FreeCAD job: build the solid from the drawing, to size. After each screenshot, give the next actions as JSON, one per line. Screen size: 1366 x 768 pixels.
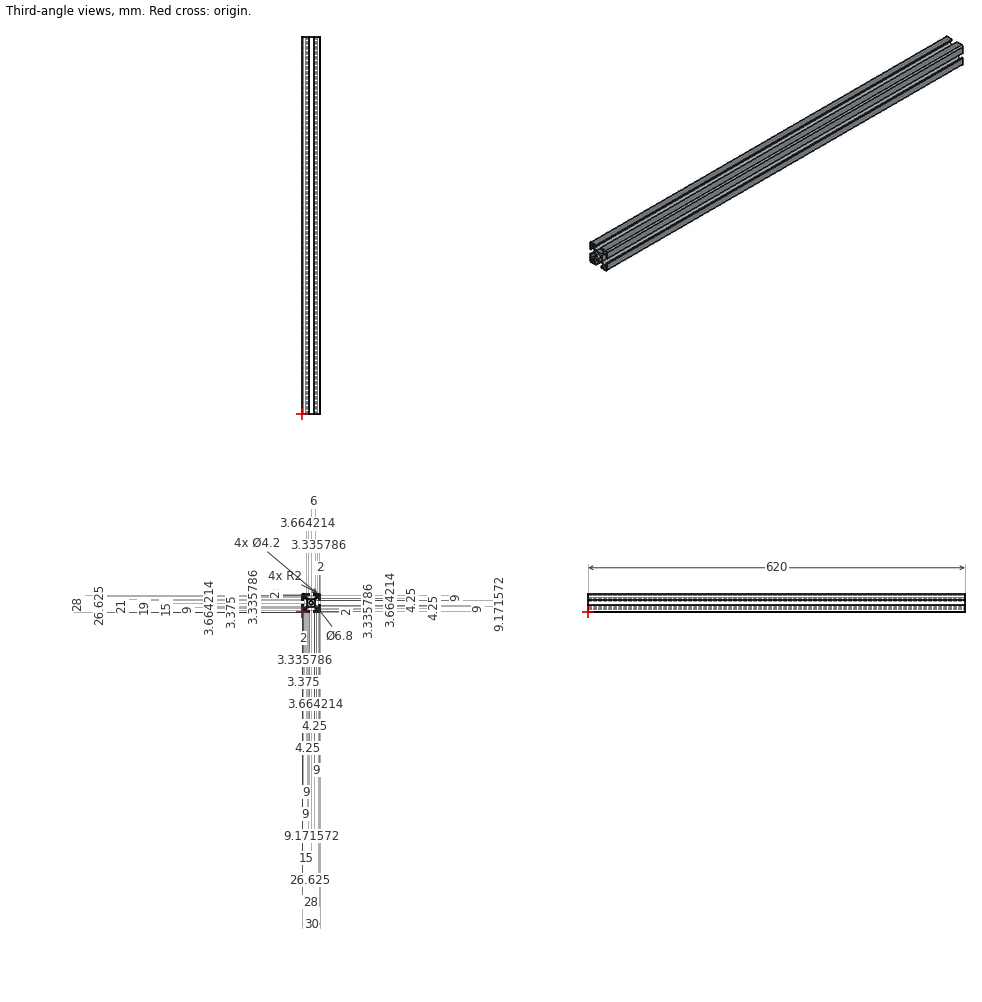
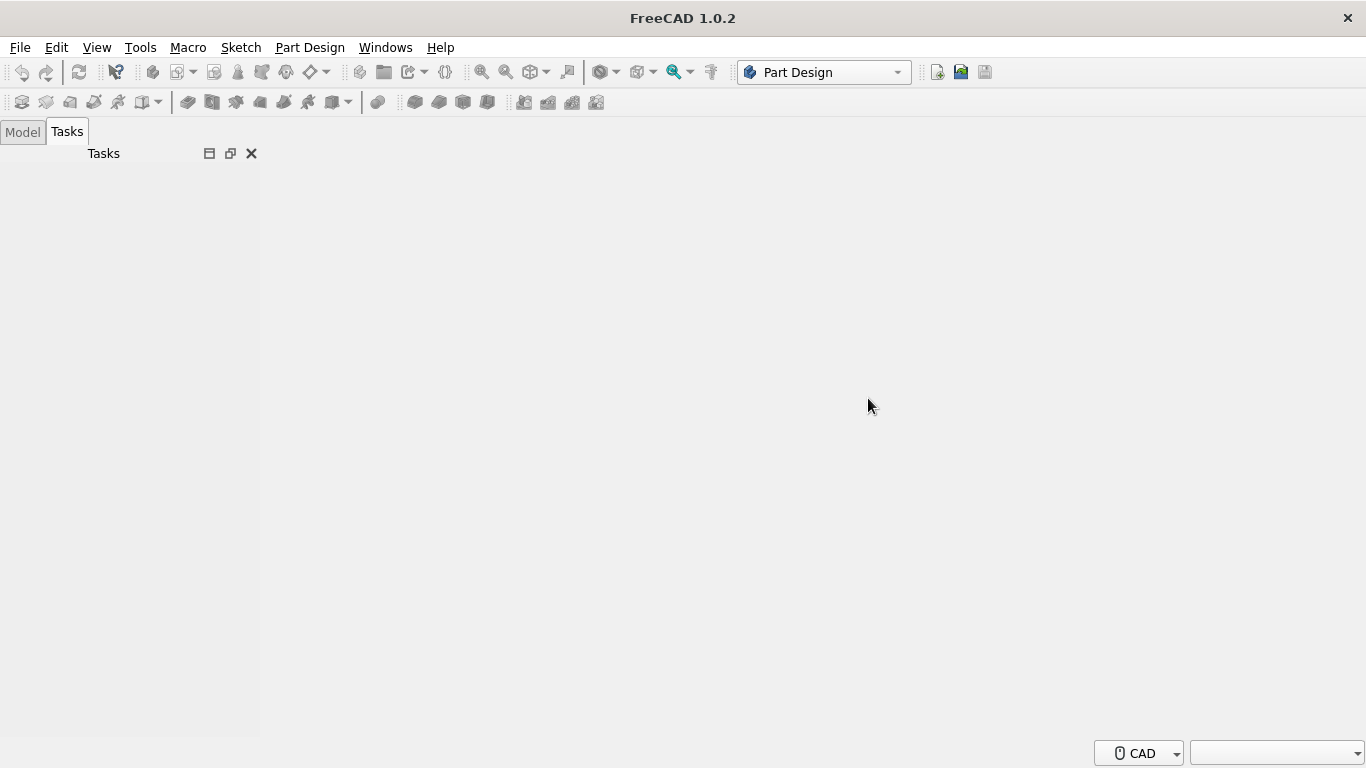
{"action": "left_click", "coordinate": [938, 72]}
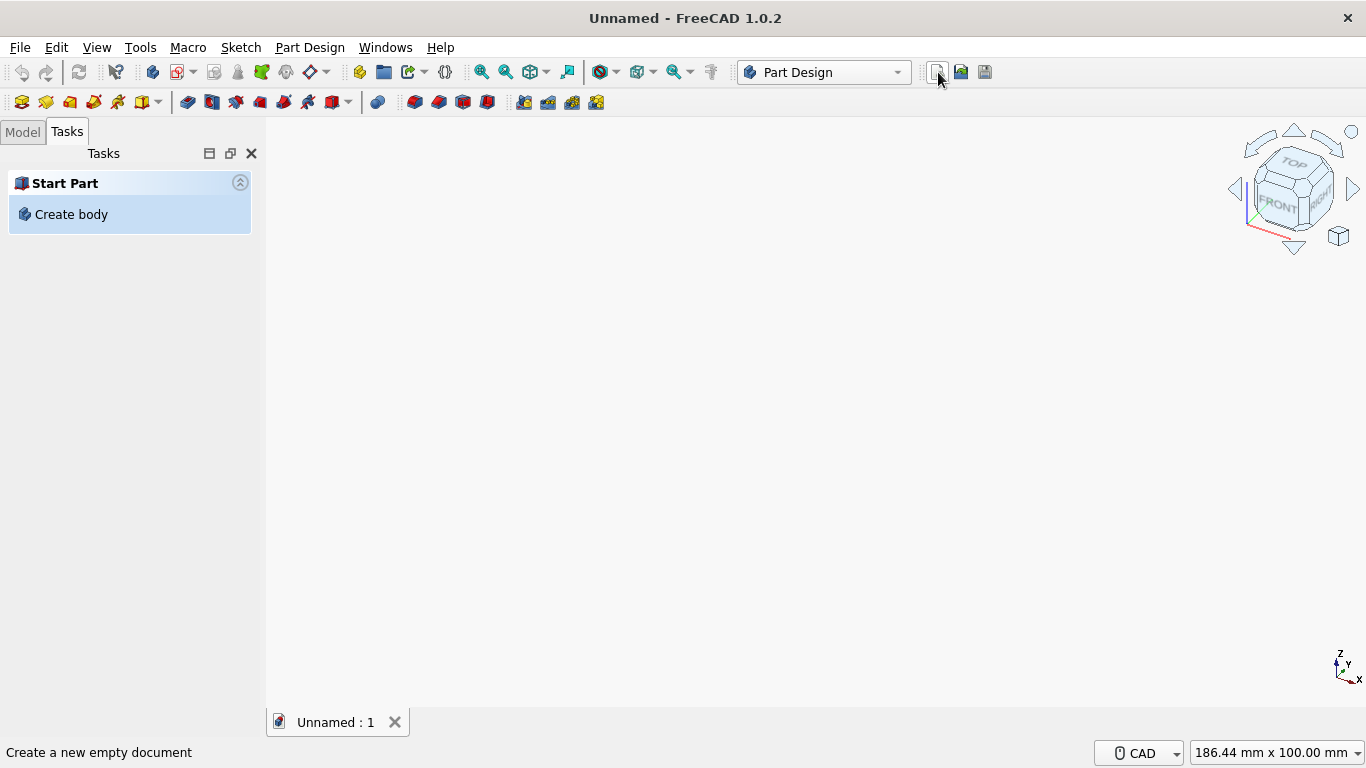
{"action": "left_click", "coordinate": [178, 72]}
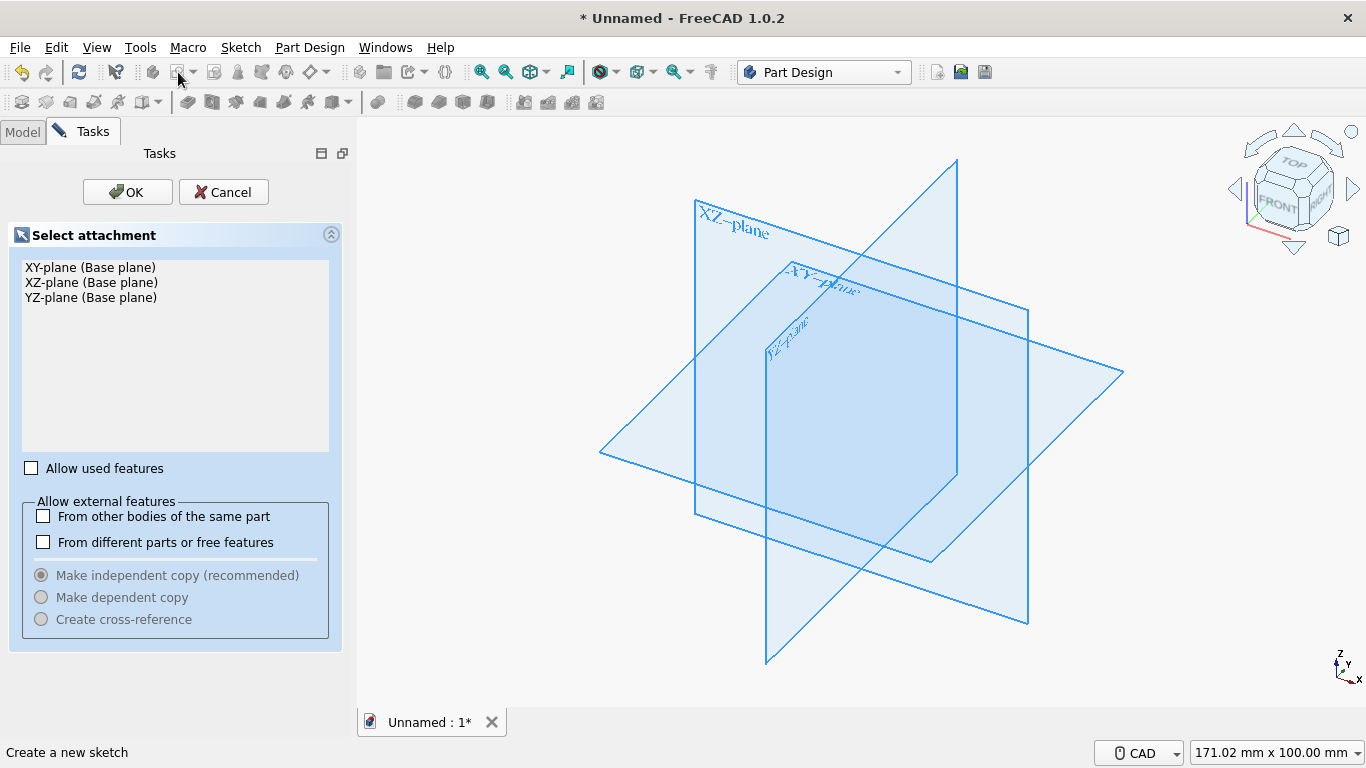
{"action": "left_click", "coordinate": [82, 282]}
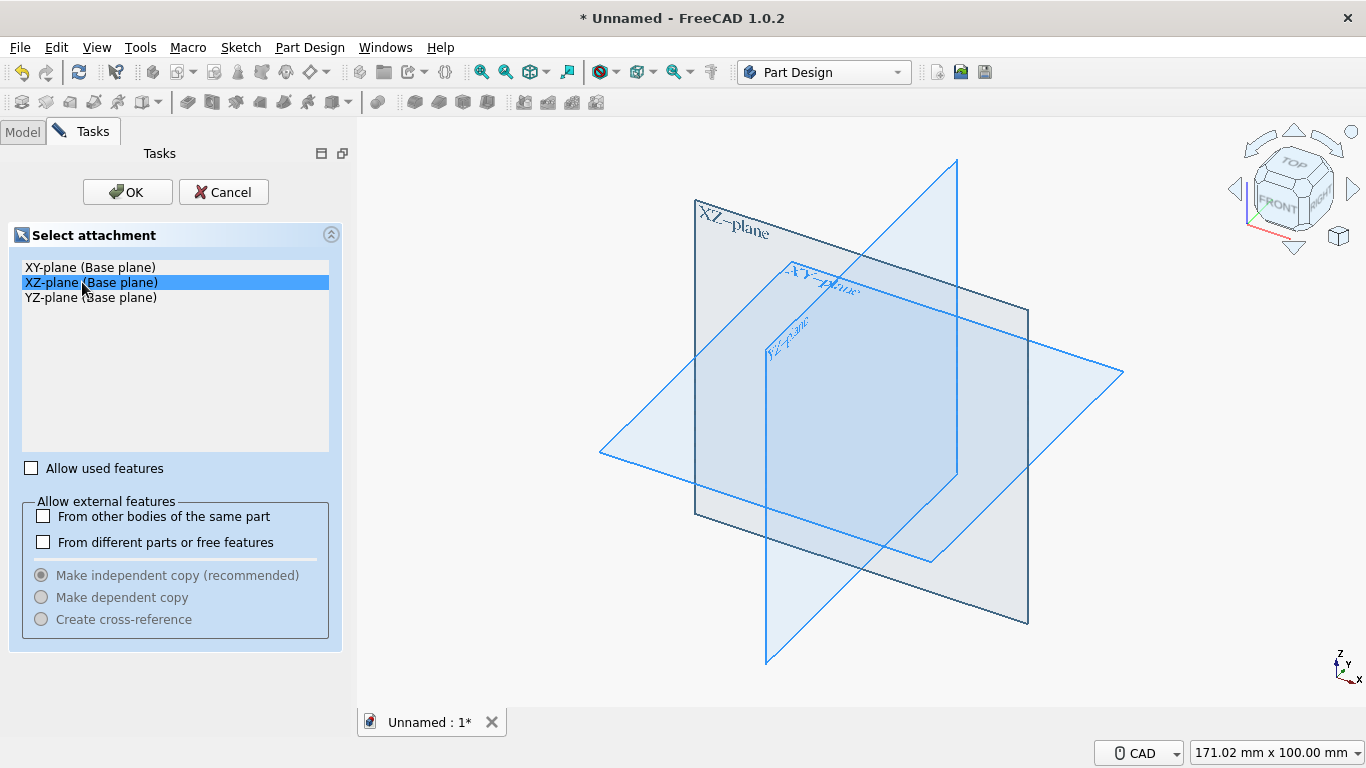
{"action": "left_click", "coordinate": [128, 192]}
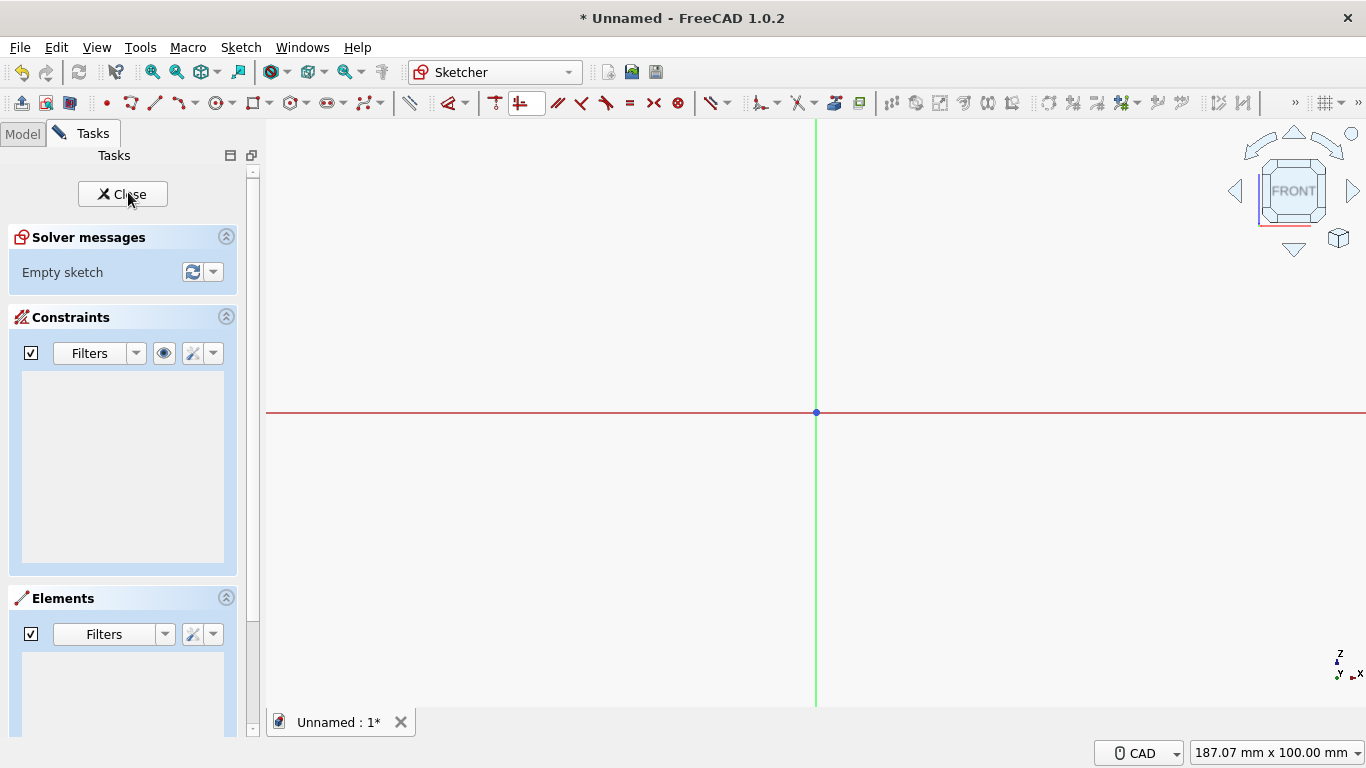
{"action": "scroll", "coordinate": [1032, 253], "scroll_direction": "up", "scroll_amount": 4}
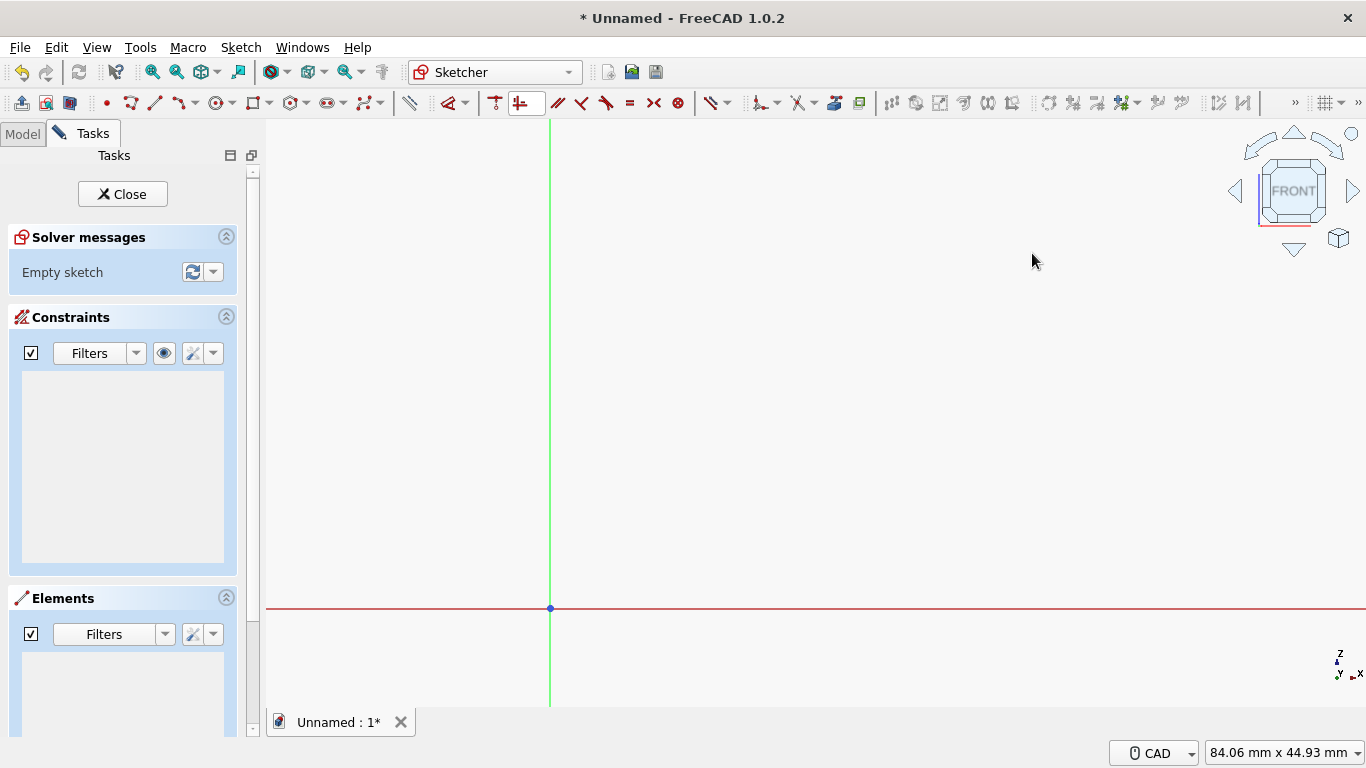
{"action": "left_click", "coordinate": [132, 104]}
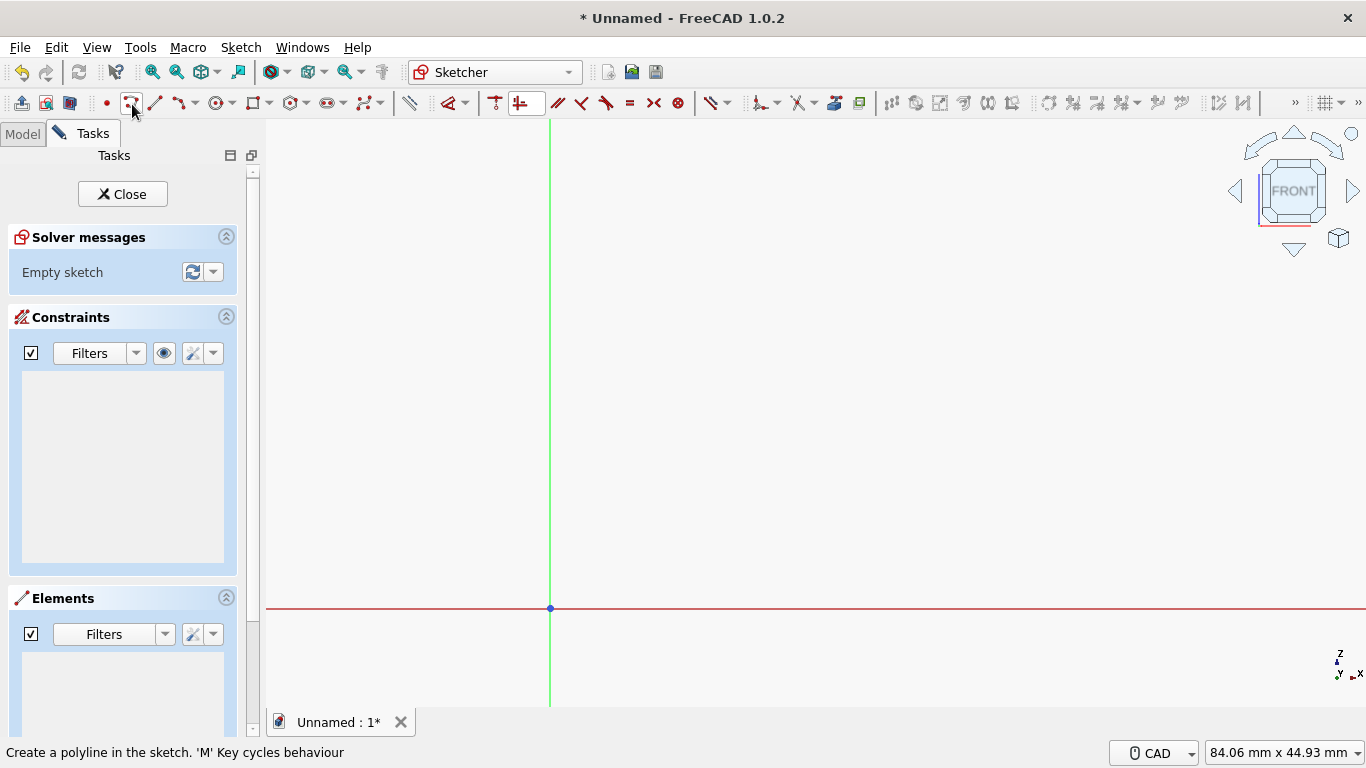
{"action": "left_click", "coordinate": [943, 242]}
{"action": "left_click", "coordinate": [943, 360]}
{"action": "left_click", "coordinate": [917, 360]}
{"action": "left_click", "coordinate": [917, 305]}
{"action": "left_click", "coordinate": [873, 305]}
{"action": "left_click", "coordinate": [825, 353]}
{"action": "left_click", "coordinate": [825, 473]}
{"action": "left_click", "coordinate": [873, 520]}
{"action": "left_click", "coordinate": [917, 520]}
{"action": "left_click", "coordinate": [917, 465]}
{"action": "left_click", "coordinate": [943, 465]}
{"action": "left_click", "coordinate": [943, 583]}
{"action": "right_click", "coordinate": [943, 583]}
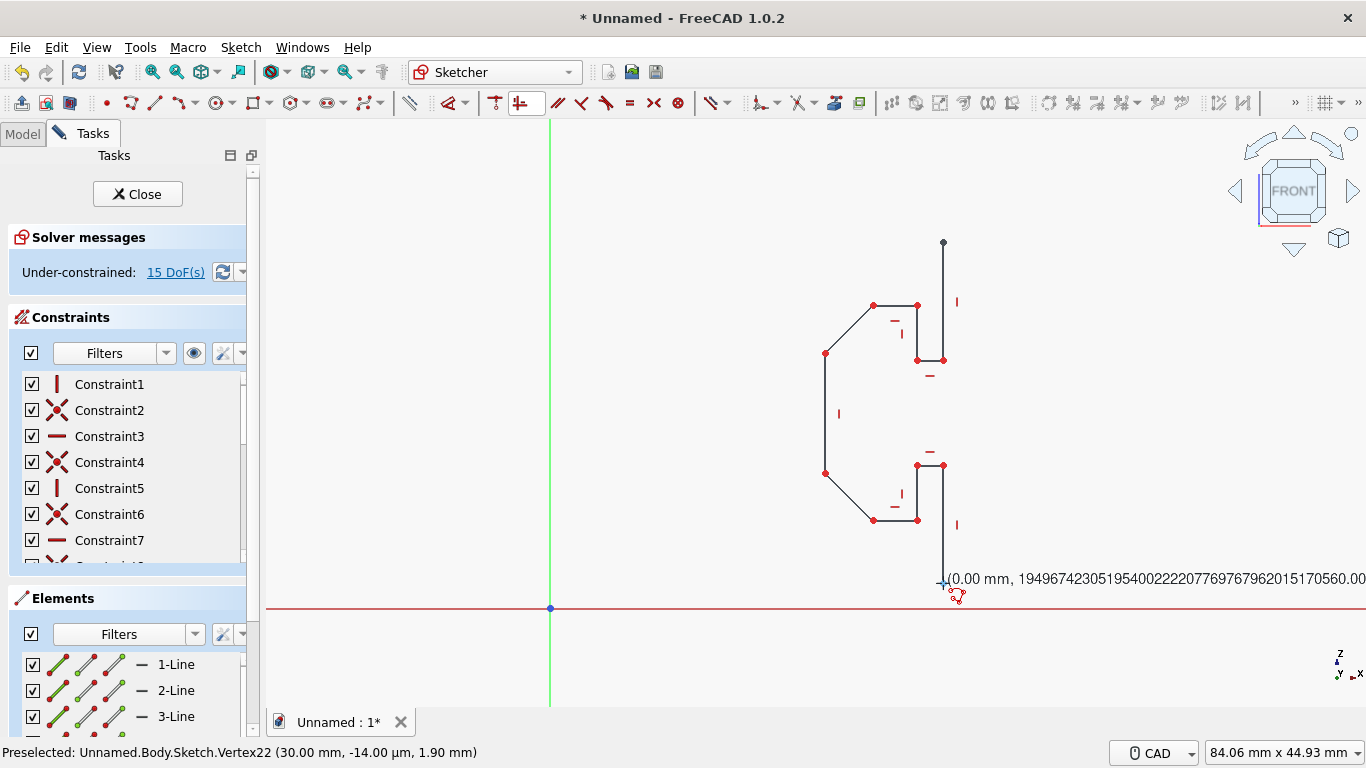
{"action": "left_click", "coordinate": [917, 609]}
{"action": "left_click", "coordinate": [799, 600]}
{"action": "left_click", "coordinate": [799, 583]}
{"action": "left_click", "coordinate": [855, 583]}
{"action": "left_click", "coordinate": [855, 539]}
{"action": "left_click", "coordinate": [807, 491]}
{"action": "left_click", "coordinate": [687, 491]}
{"action": "left_click", "coordinate": [639, 539]}
{"action": "left_click", "coordinate": [639, 583]}
{"action": "left_click", "coordinate": [694, 583]}
{"action": "left_click", "coordinate": [694, 609]}
{"action": "left_click", "coordinate": [577, 600]}
{"action": "right_click", "coordinate": [577, 600]}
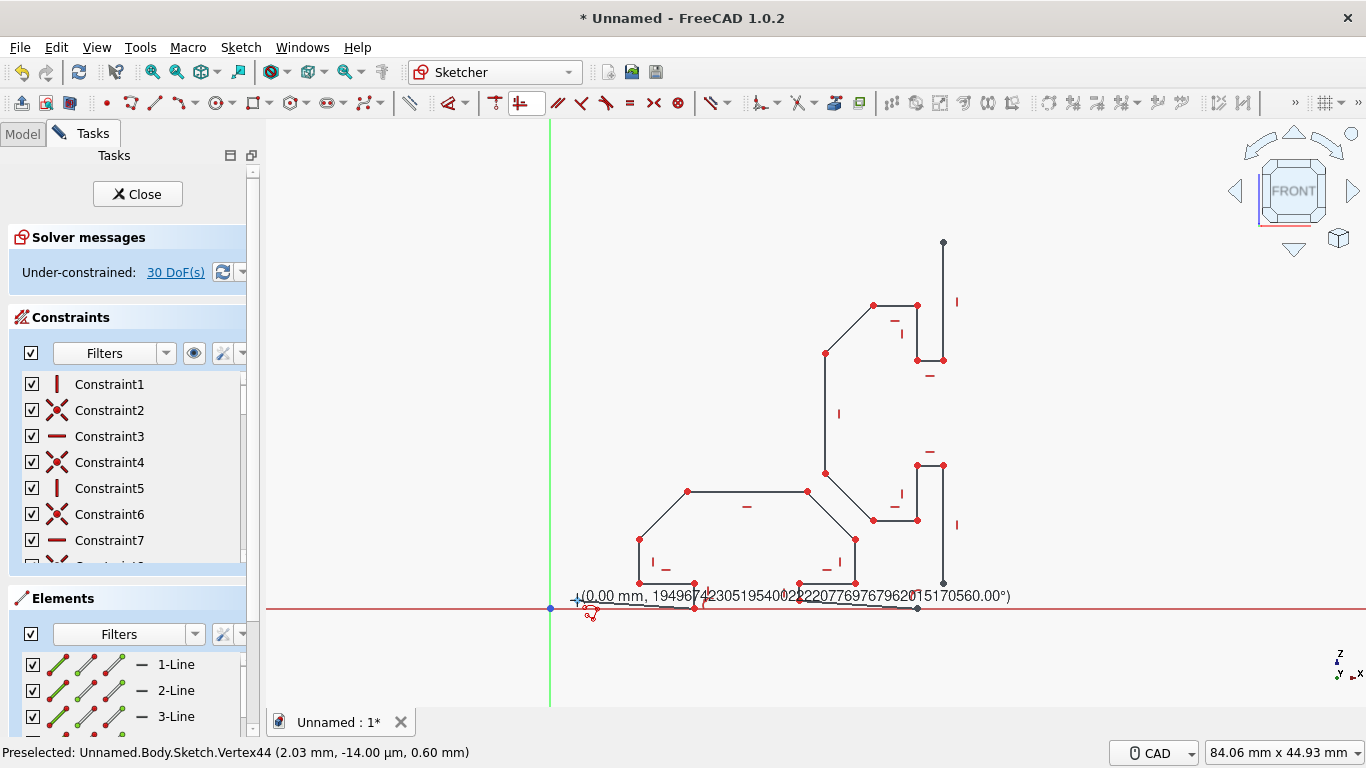
{"action": "left_click", "coordinate": [550, 583]}
{"action": "left_click", "coordinate": [559, 465]}
{"action": "left_click", "coordinate": [577, 465]}
{"action": "left_click", "coordinate": [577, 520]}
{"action": "left_click", "coordinate": [620, 520]}
{"action": "left_click", "coordinate": [668, 473]}
{"action": "left_click", "coordinate": [668, 353]}
{"action": "left_click", "coordinate": [620, 305]}
{"action": "left_click", "coordinate": [577, 305]}
{"action": "left_click", "coordinate": [577, 360]}
{"action": "left_click", "coordinate": [550, 360]}
{"action": "left_click", "coordinate": [559, 242]}
{"action": "right_click", "coordinate": [559, 242]}